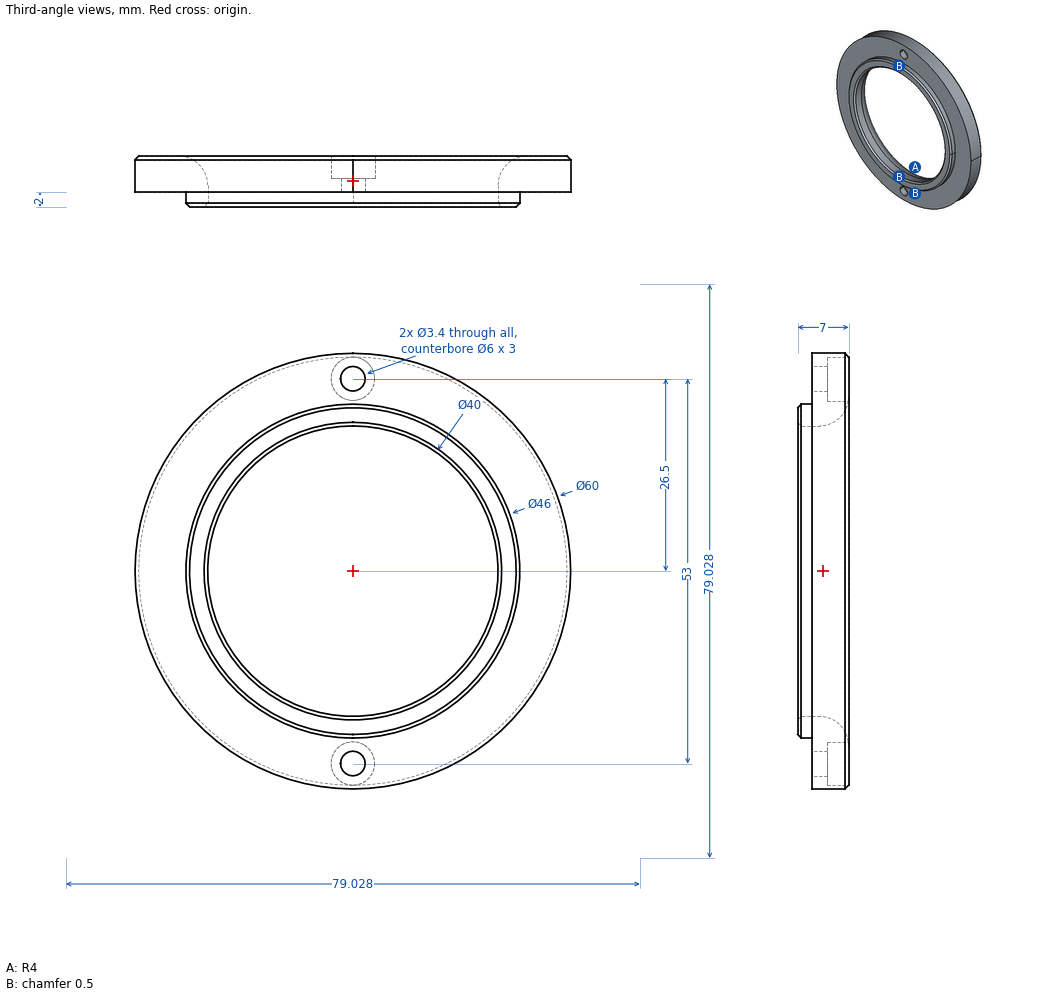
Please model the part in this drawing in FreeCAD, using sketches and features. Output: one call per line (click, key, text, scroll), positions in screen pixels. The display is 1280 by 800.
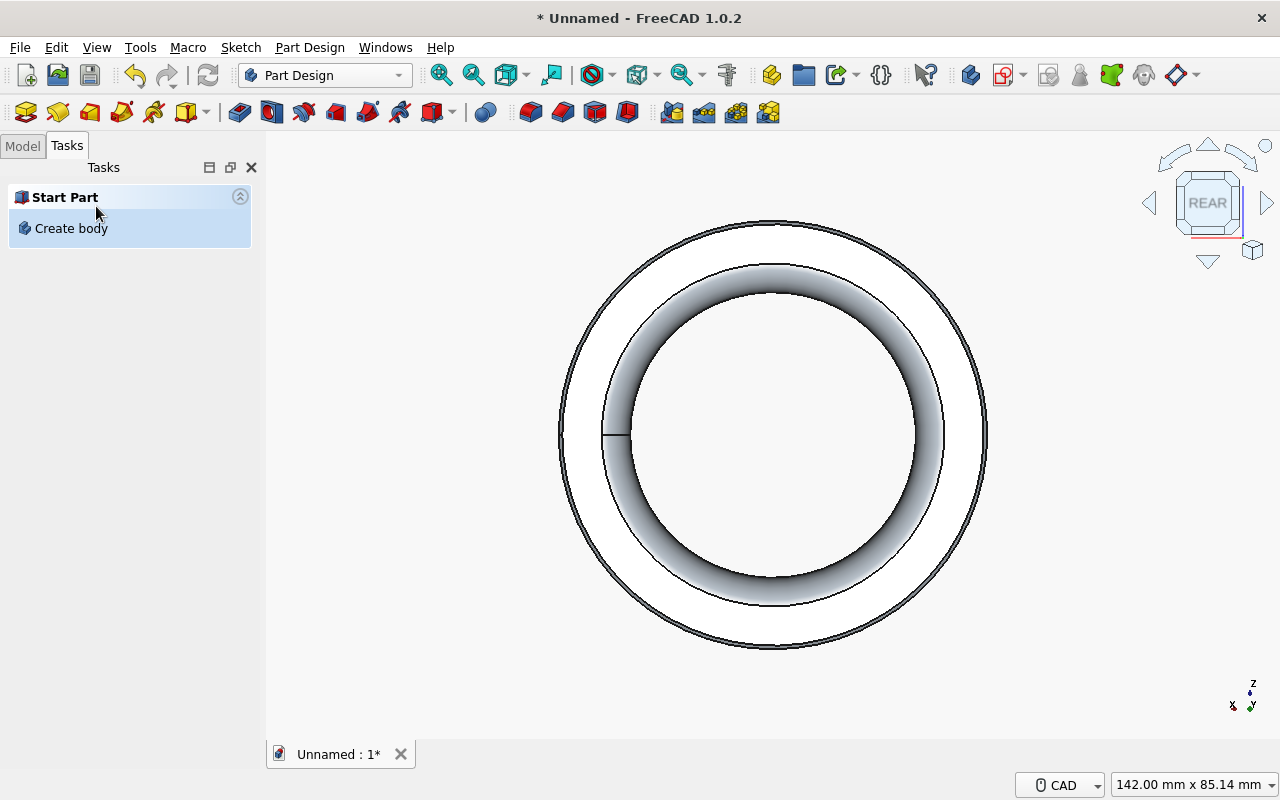
click(592, 374)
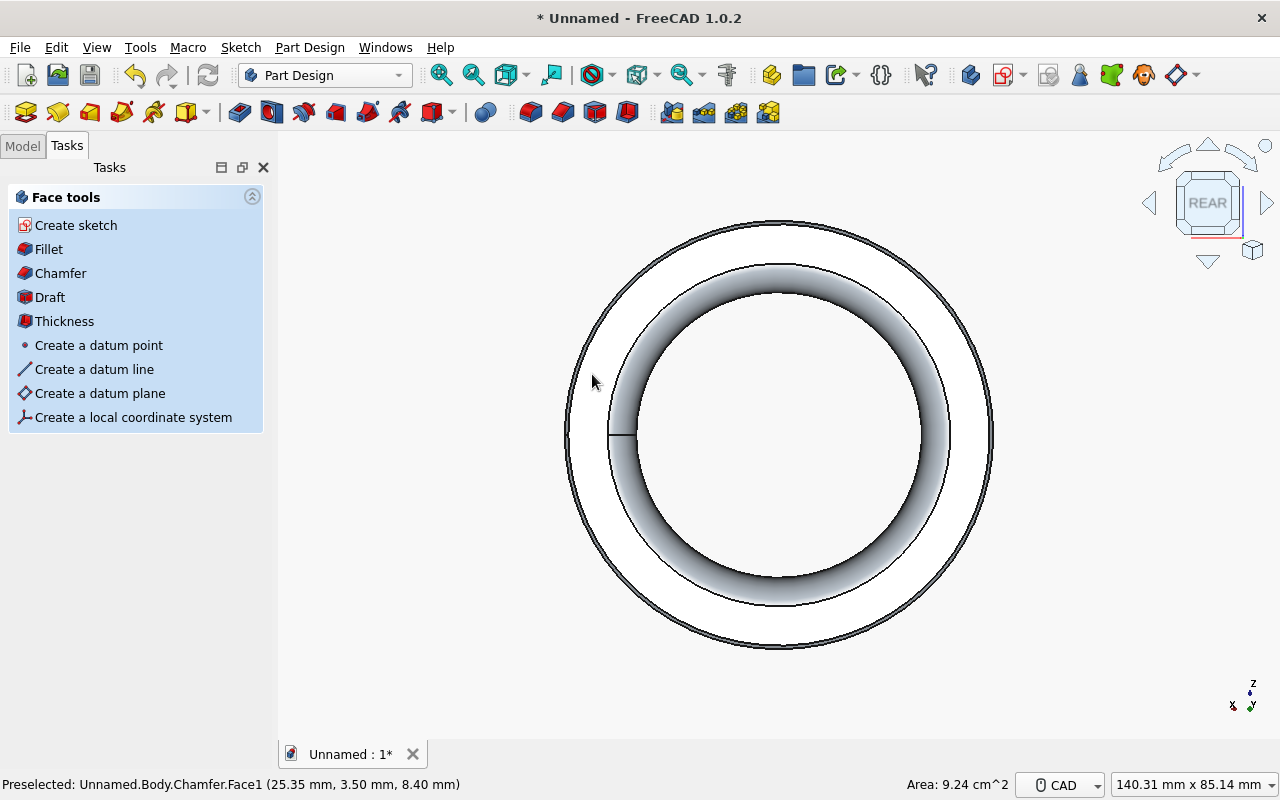
click(1004, 76)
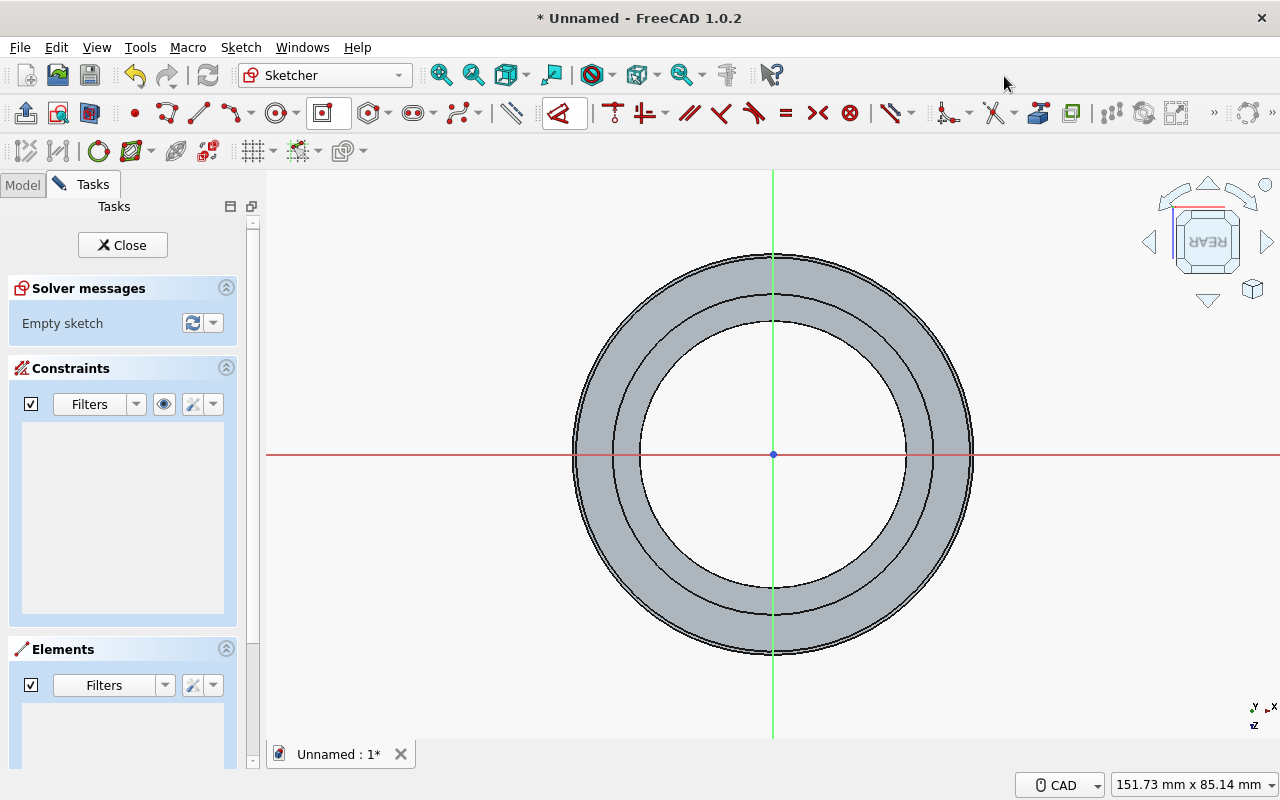
click(276, 114)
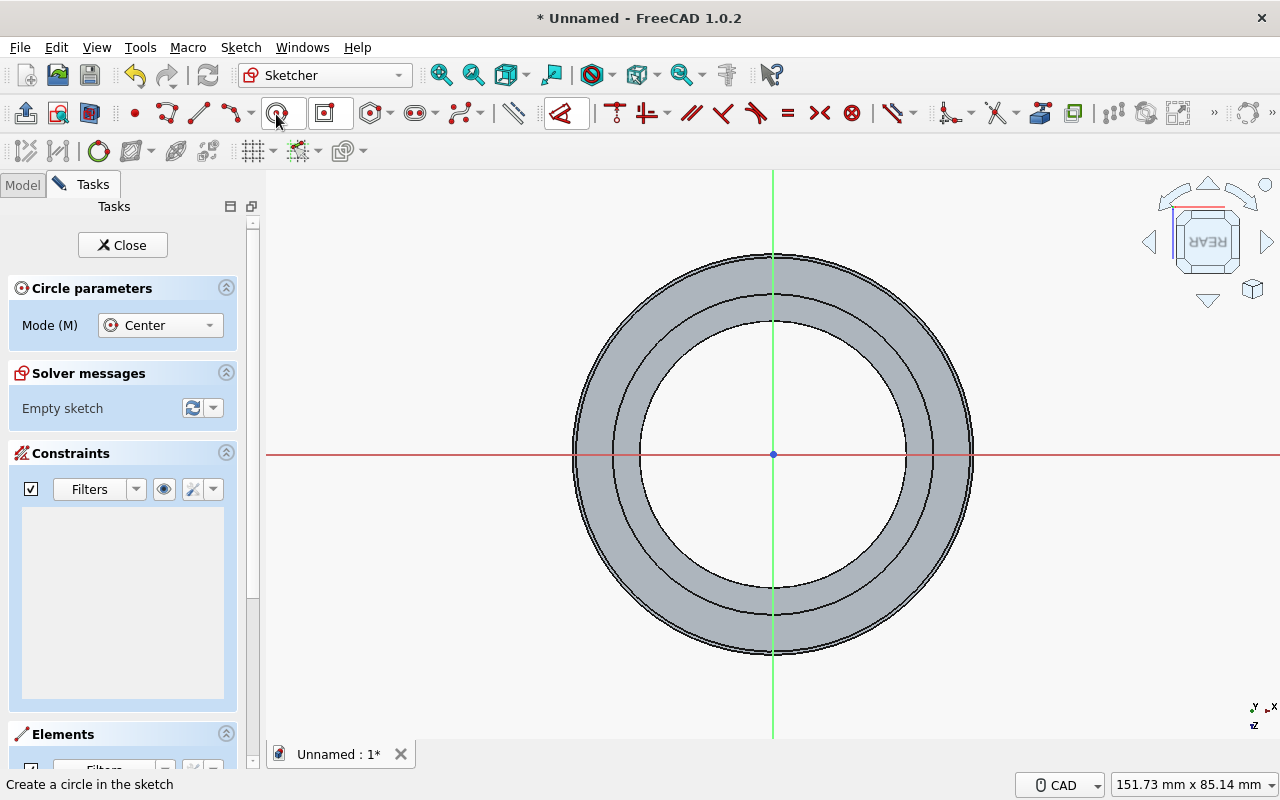
scroll(773, 632, up, 4)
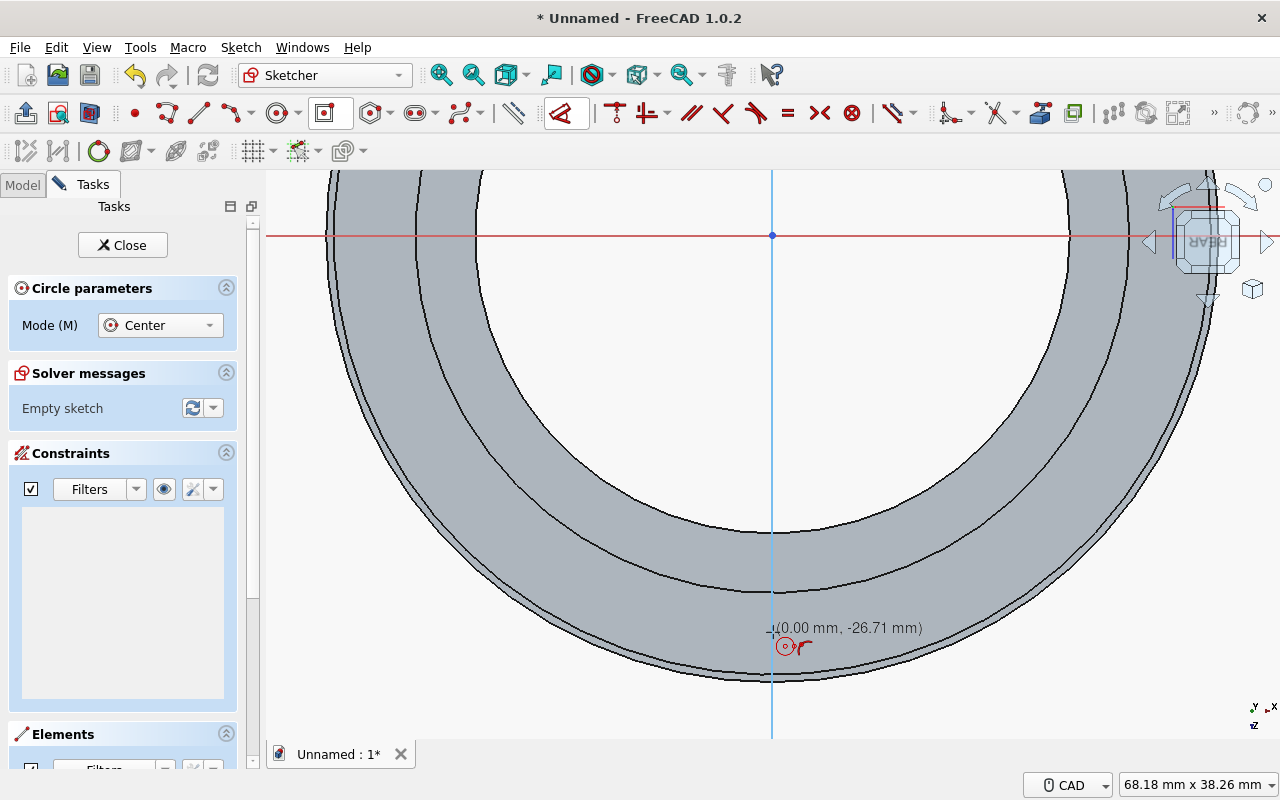
click(772, 630)
click(790, 612)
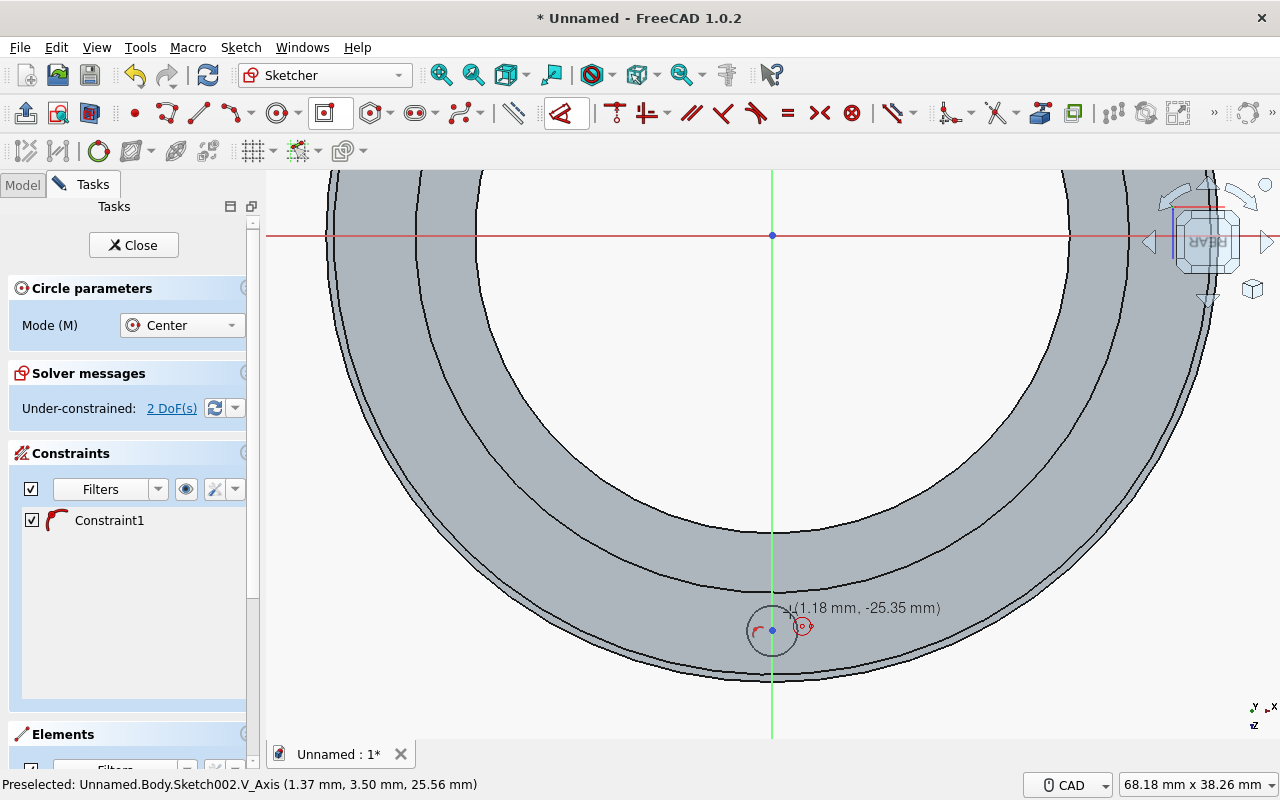
scroll(649, 633, down, 4)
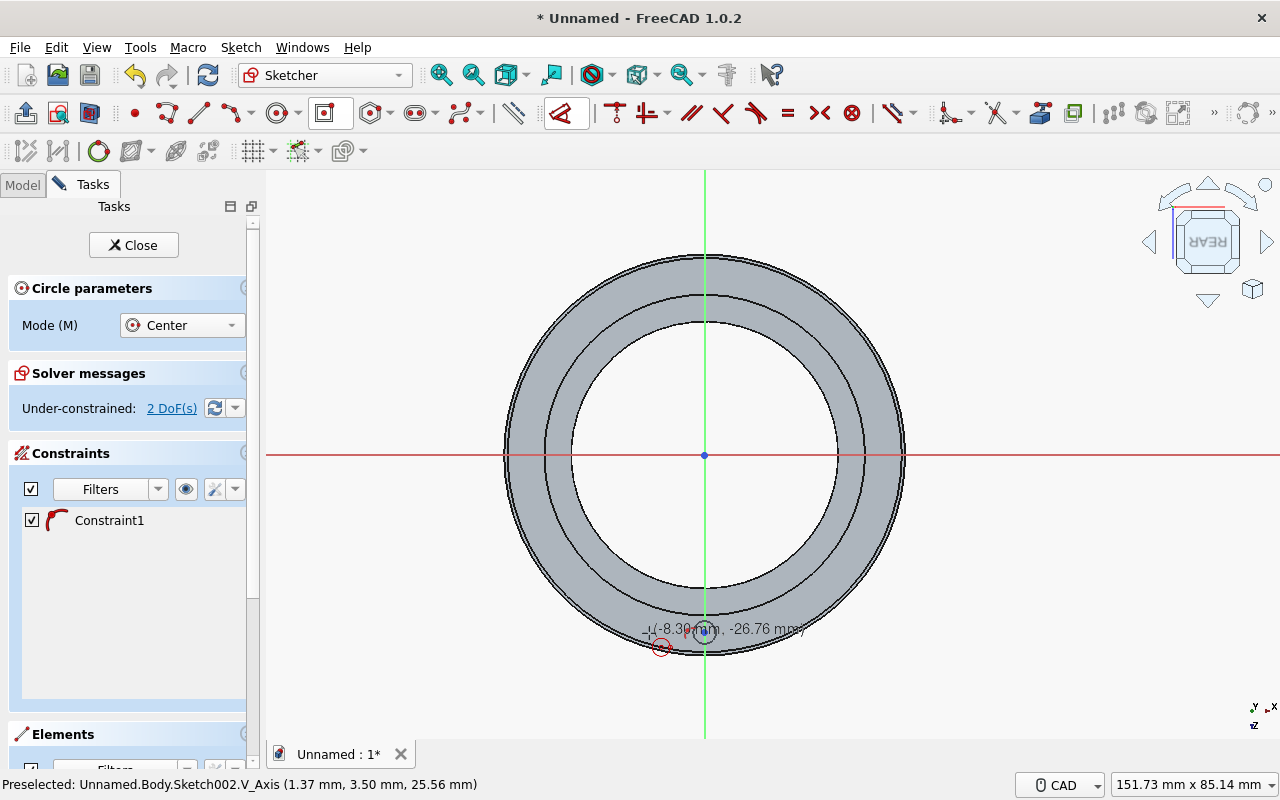
scroll(705, 278, up, 4)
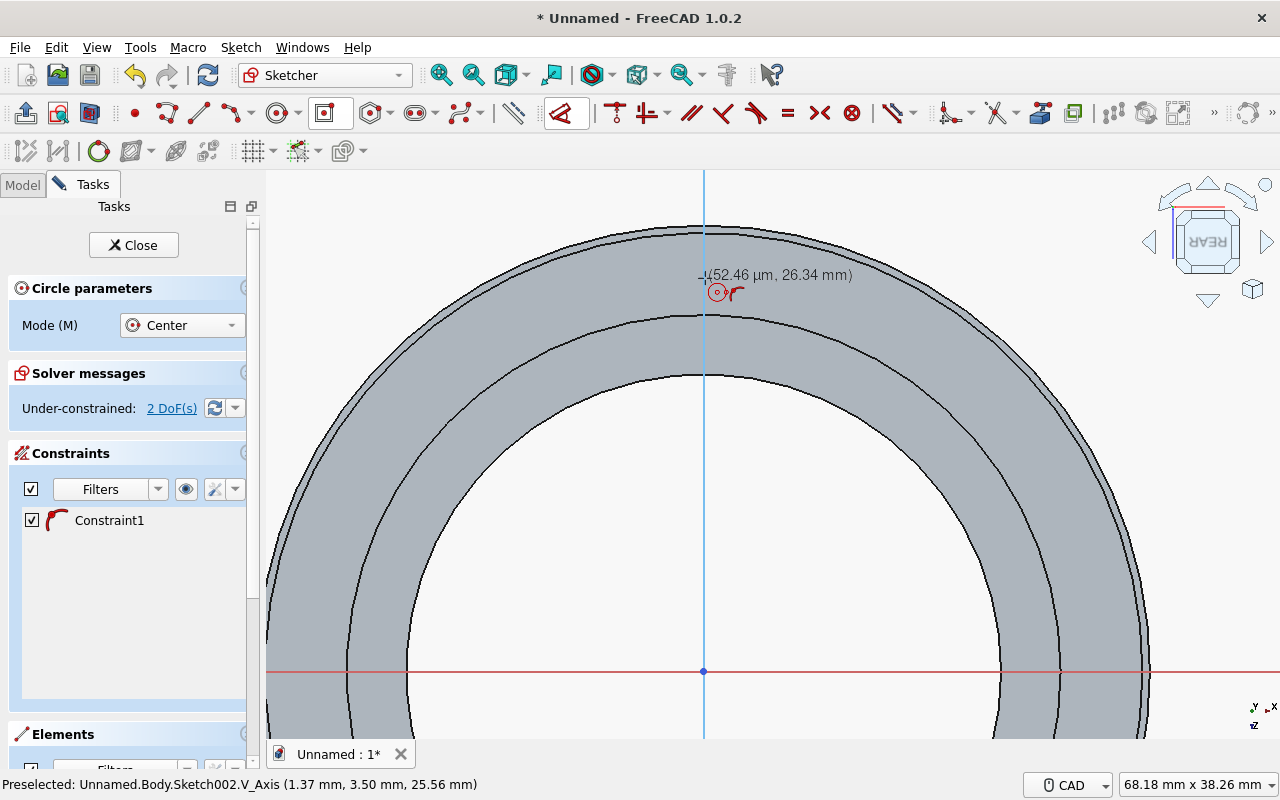
click(704, 278)
click(722, 260)
key(Escape)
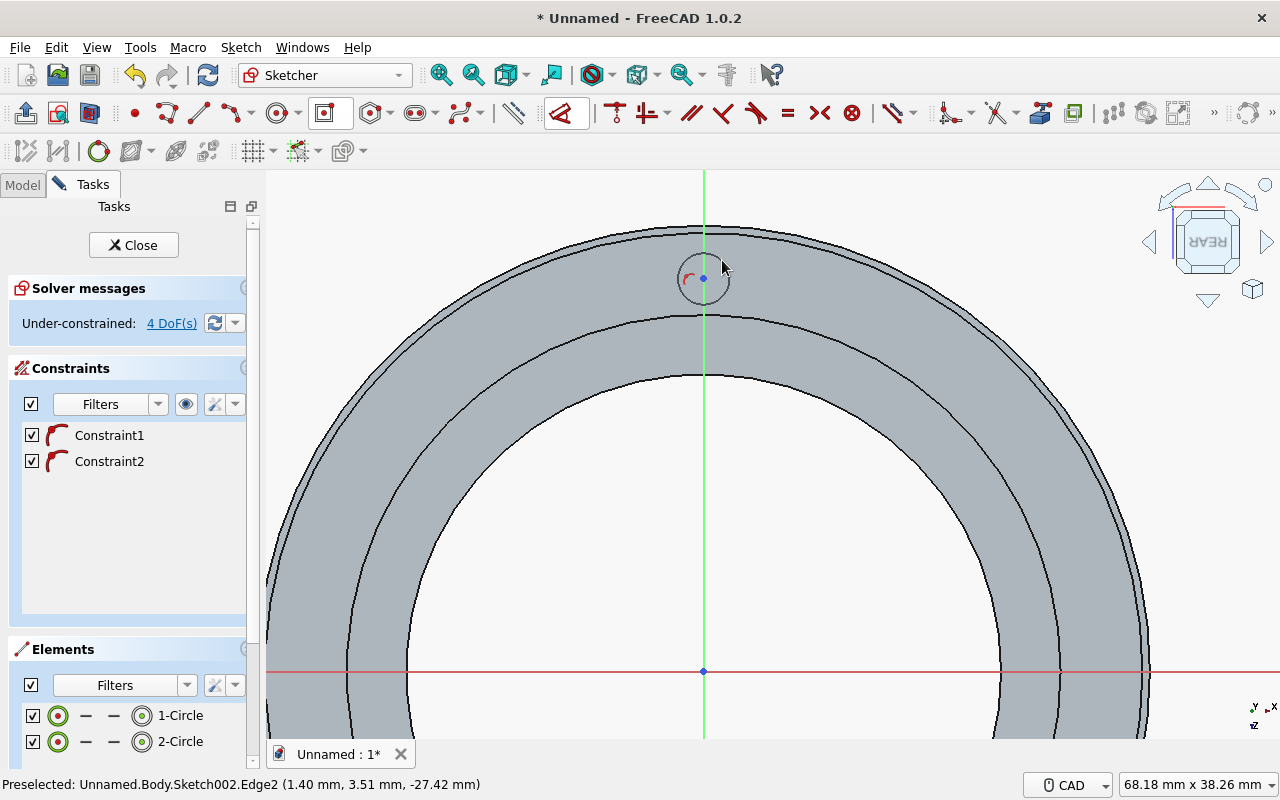
scroll(705, 277, down, 4)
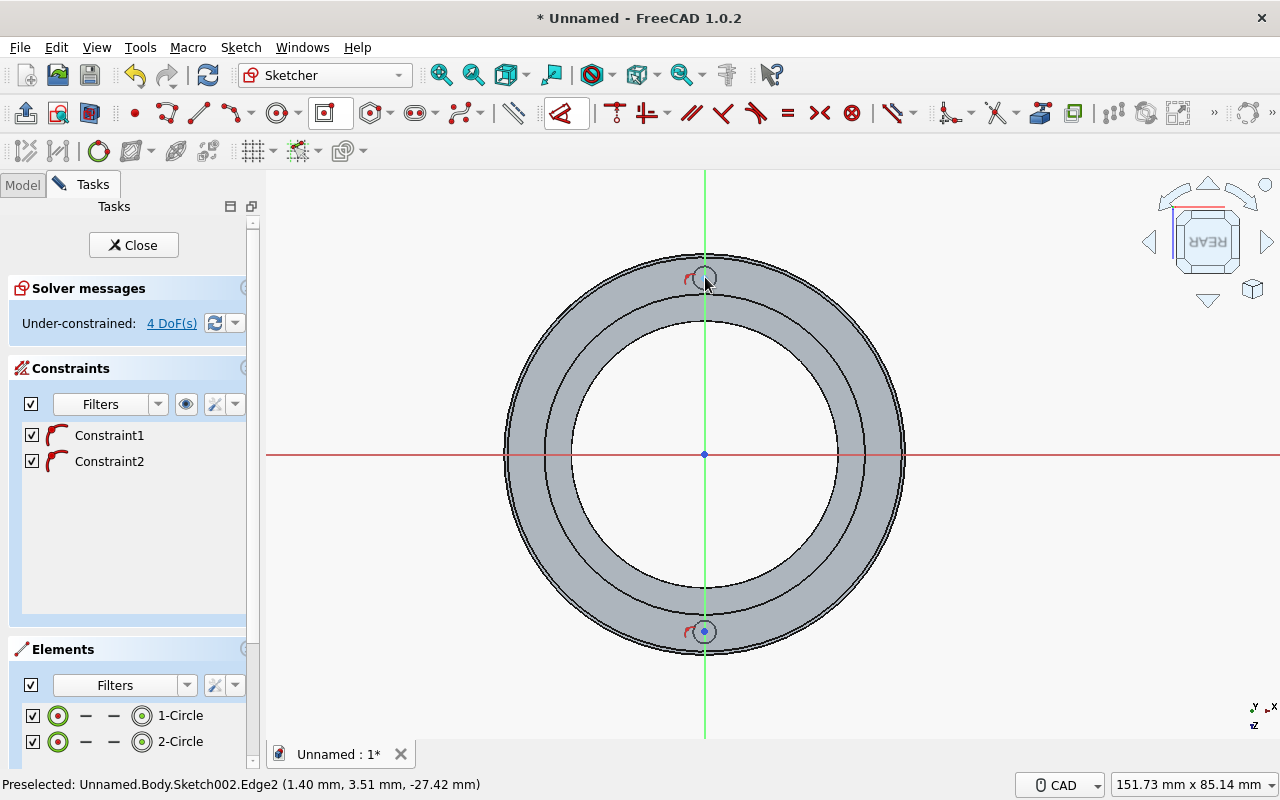
scroll(713, 624, up, 3)